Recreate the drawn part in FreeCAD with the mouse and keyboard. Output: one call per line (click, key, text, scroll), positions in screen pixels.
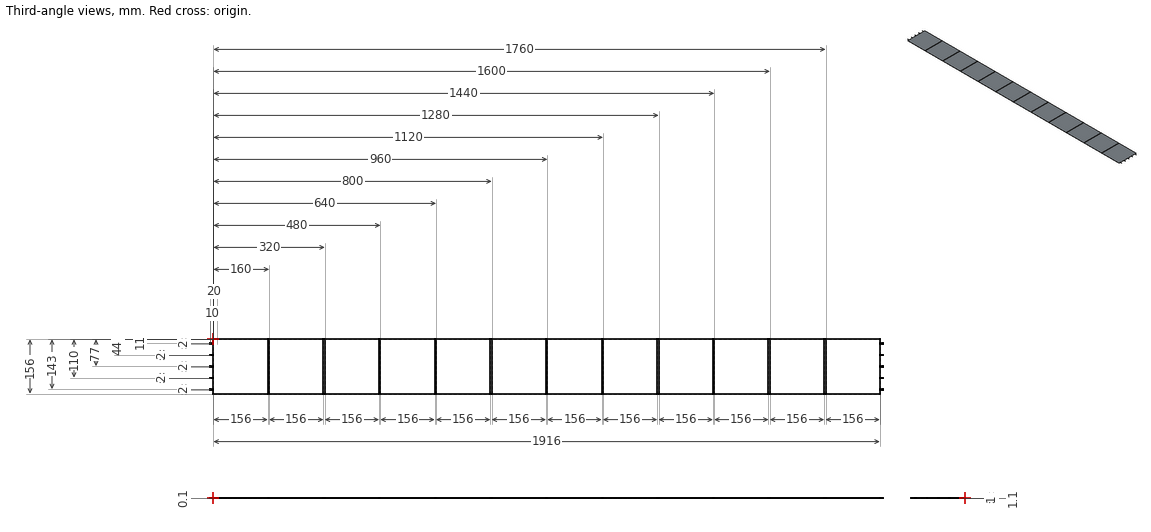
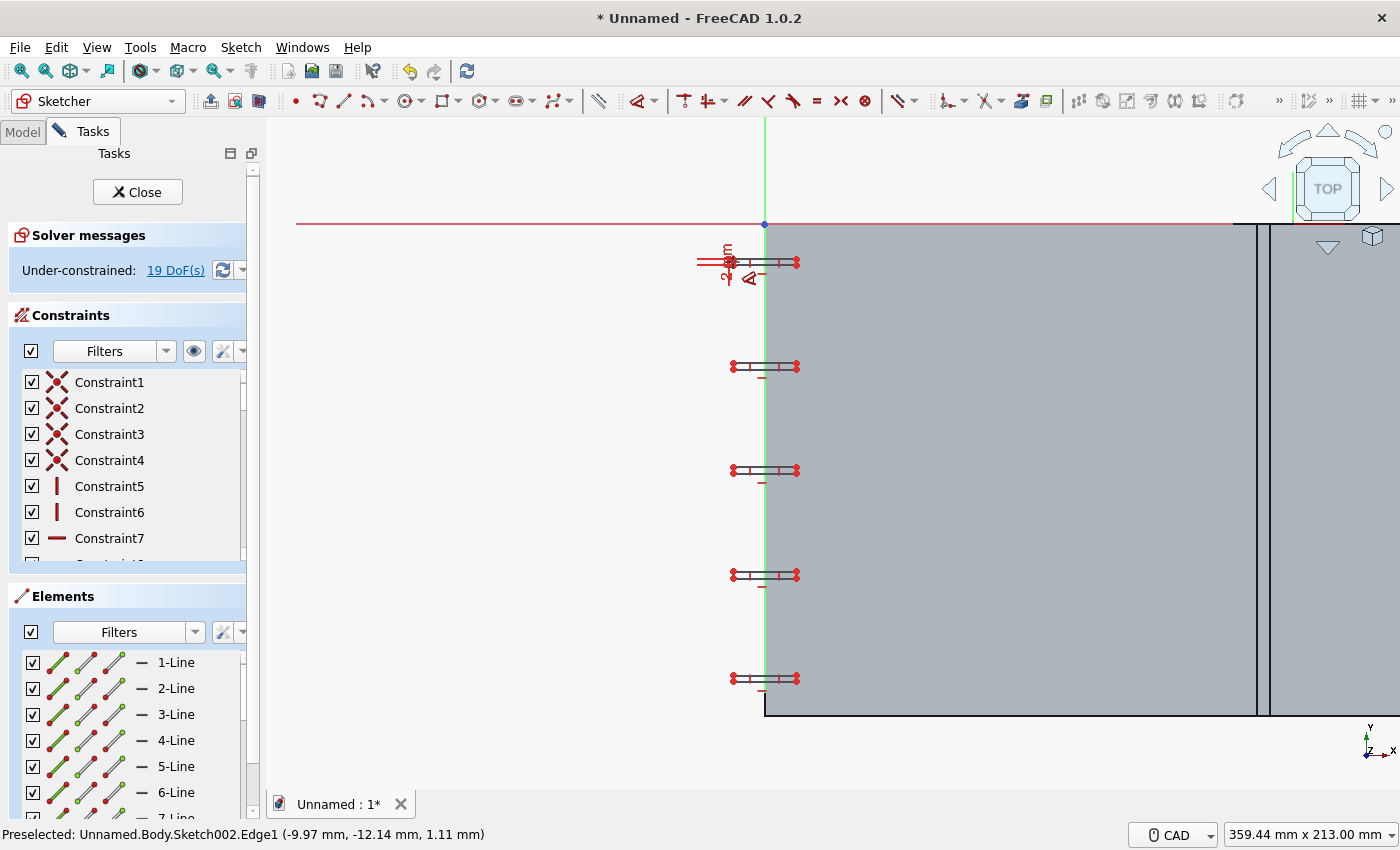
scroll(733, 365, up, 10)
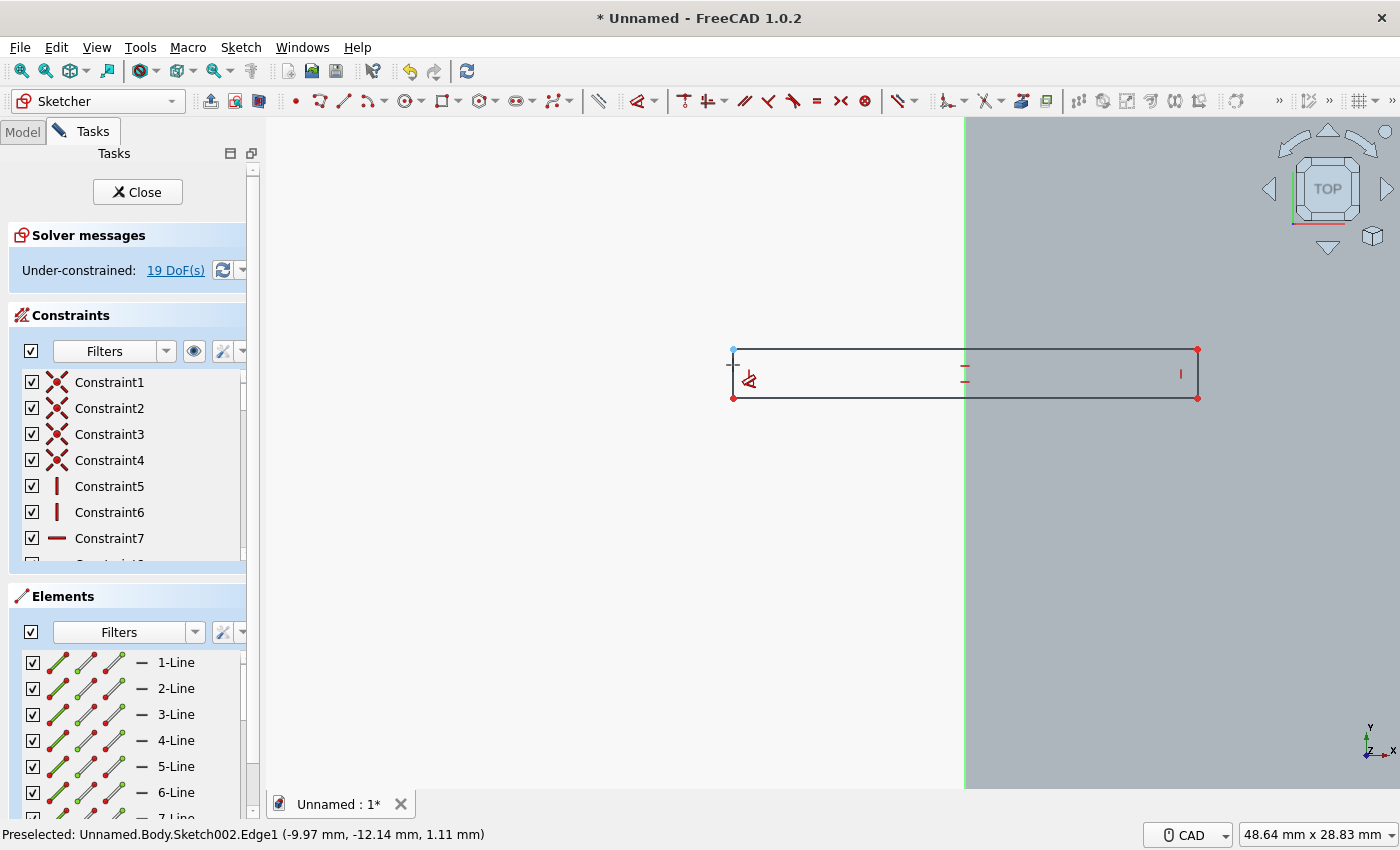
click(733, 364)
click(699, 374)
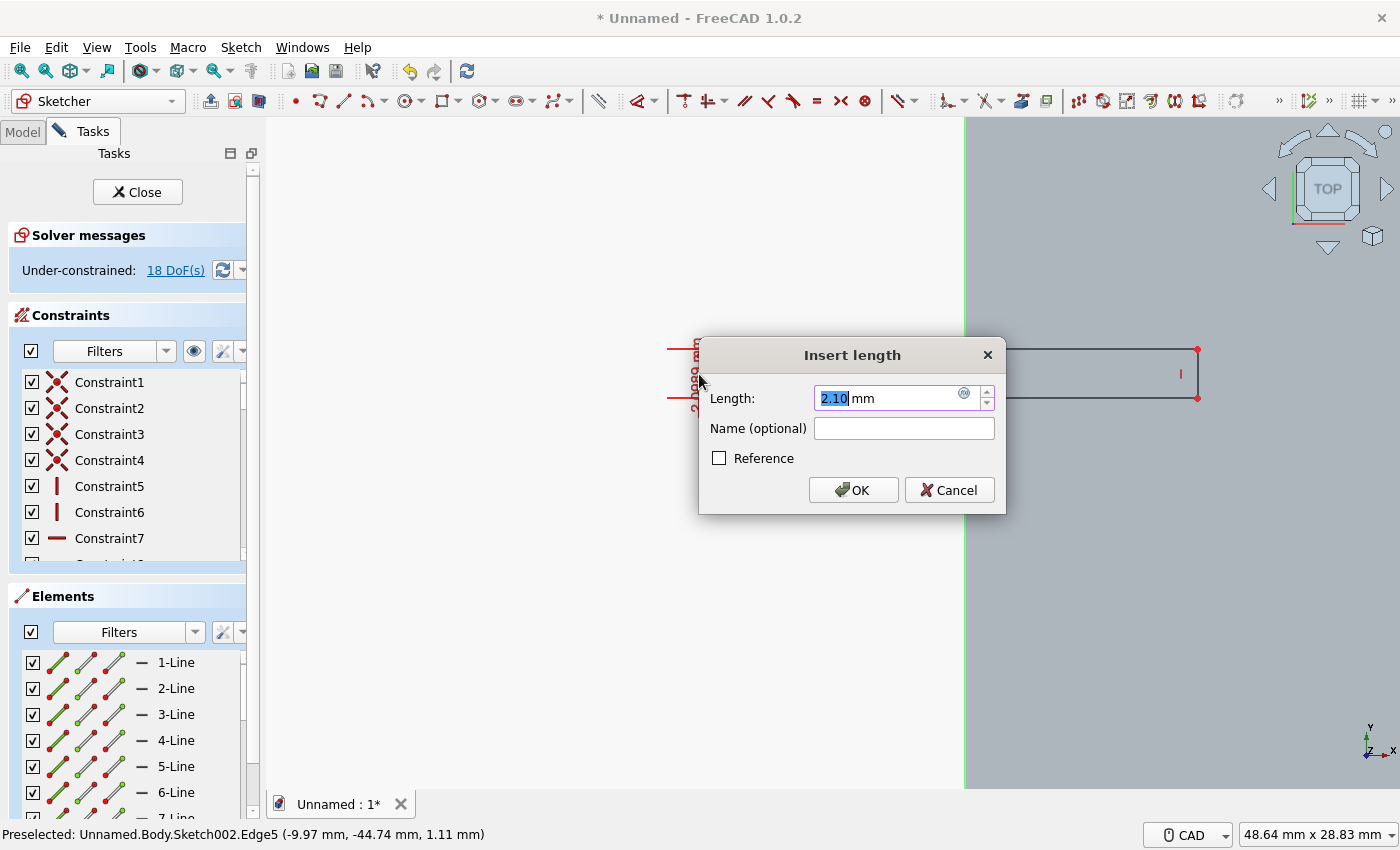
text(2)
key(Return)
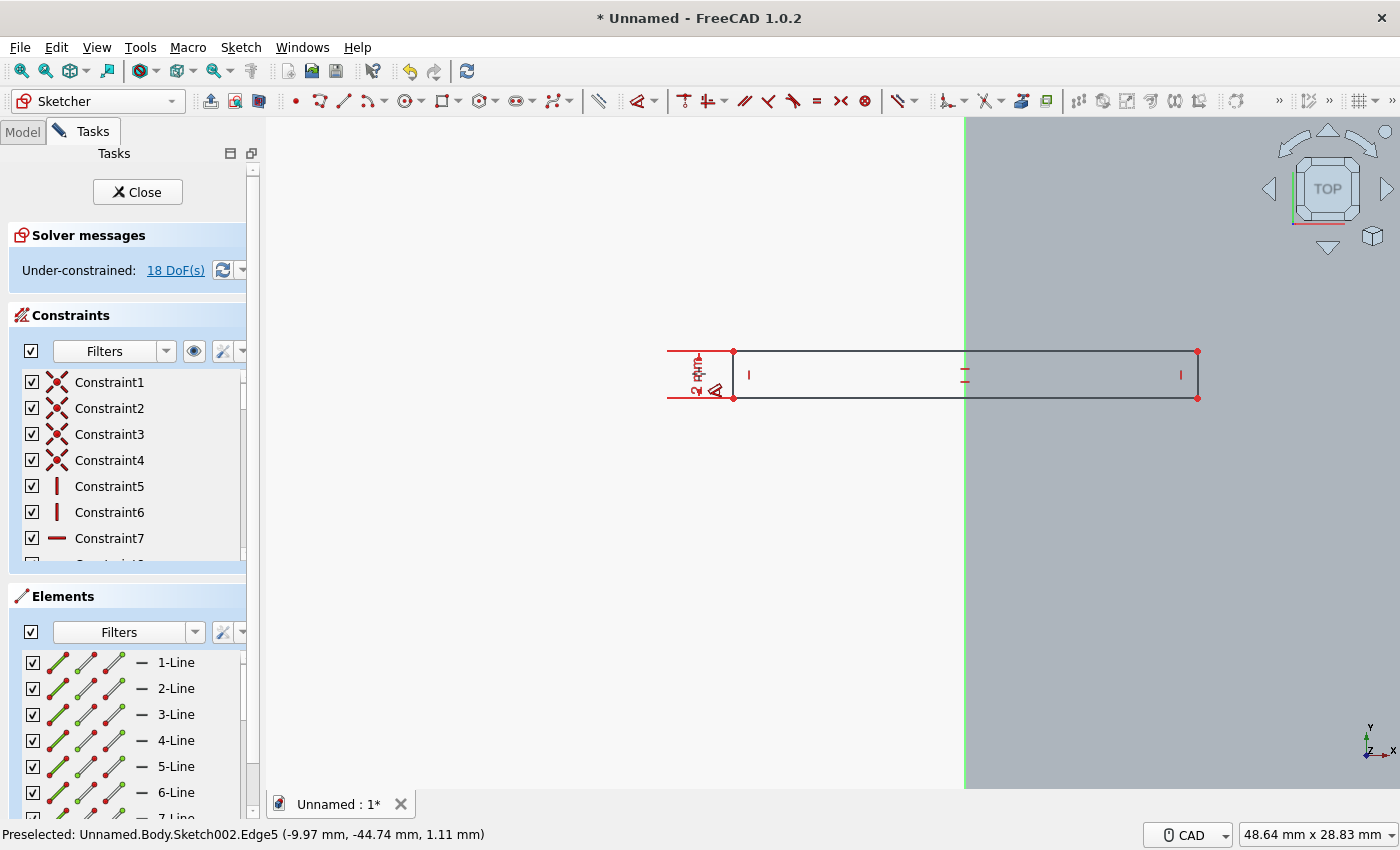
scroll(733, 365, down, 10)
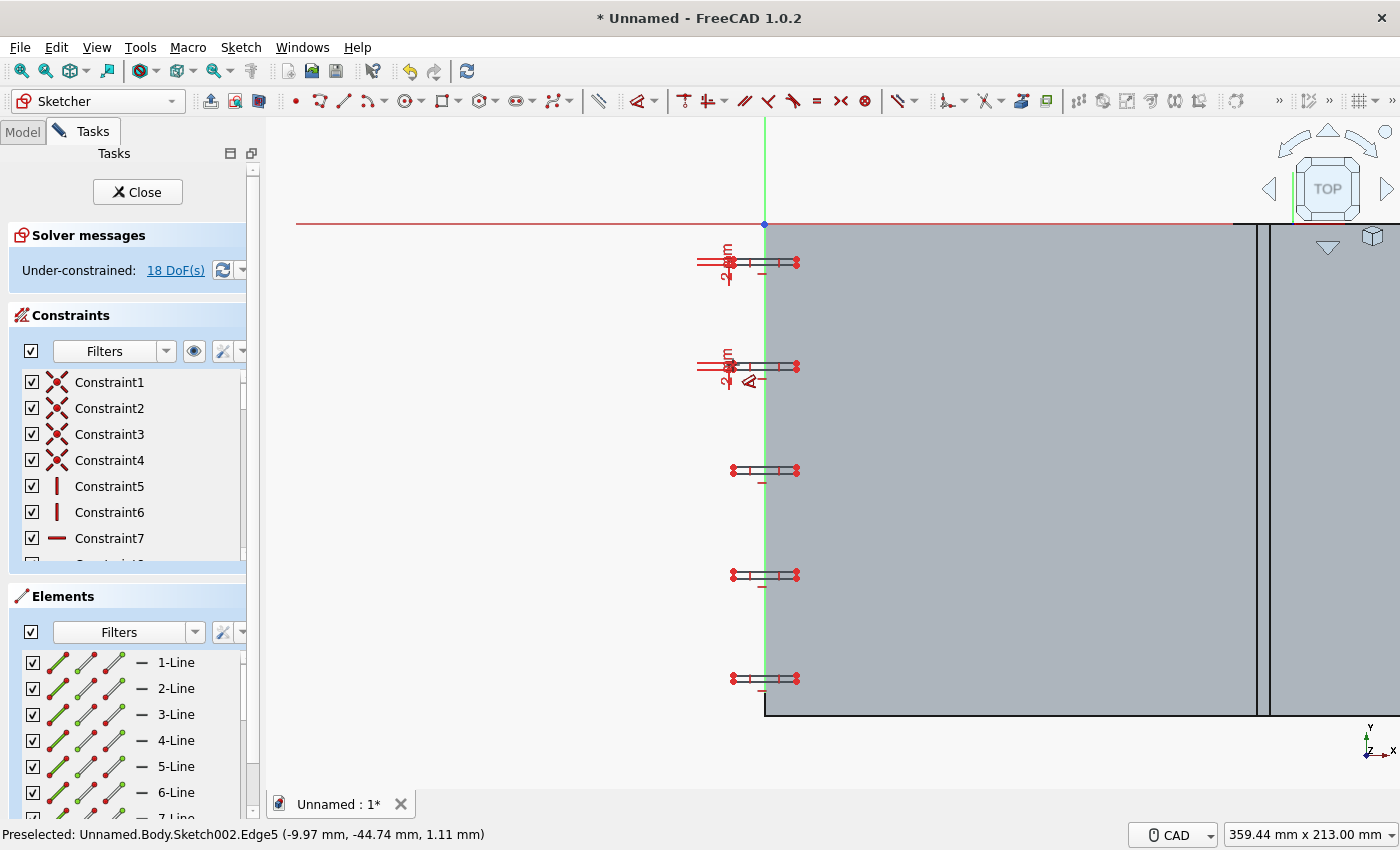
scroll(733, 469, up, 10)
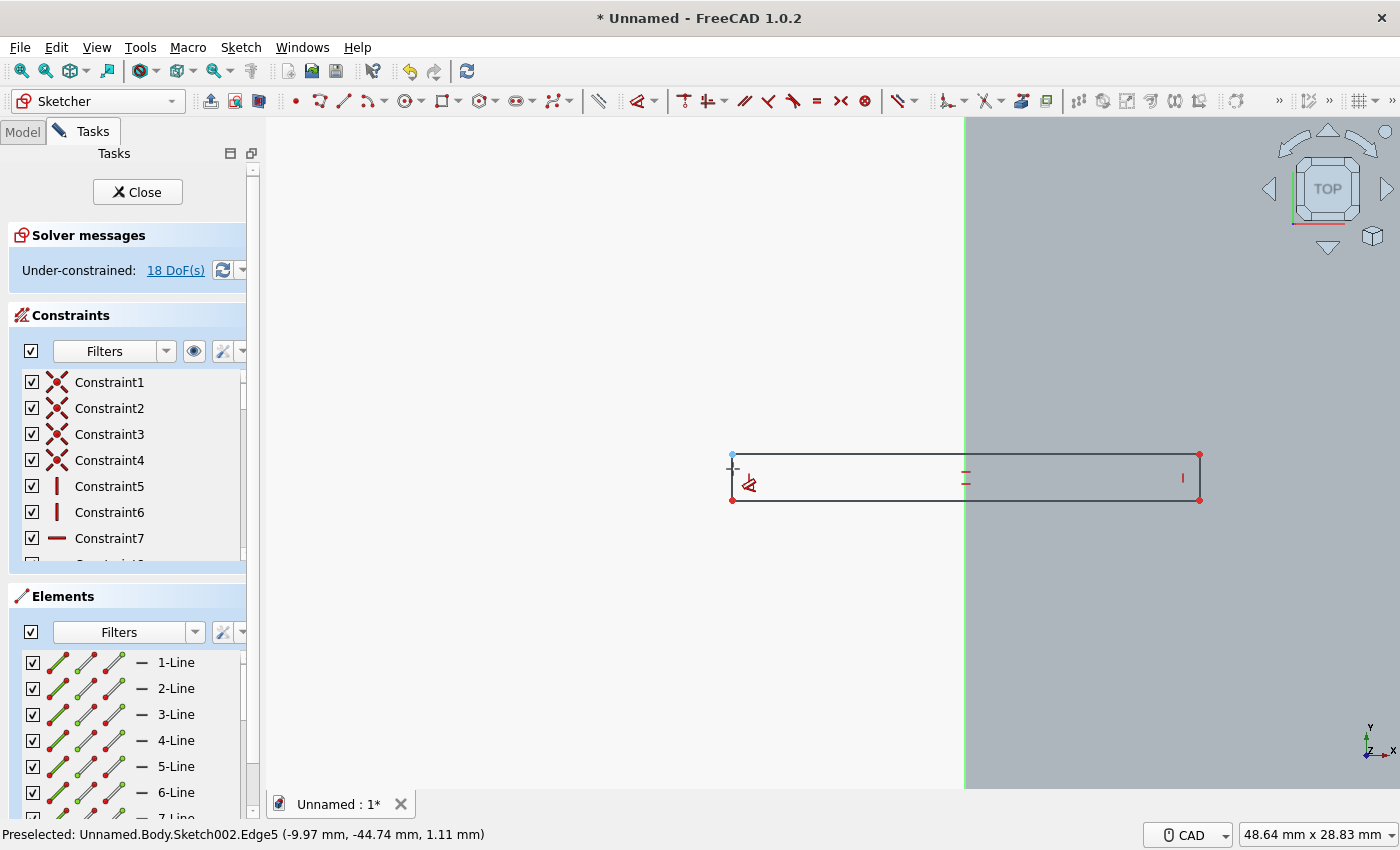
click(732, 468)
click(698, 477)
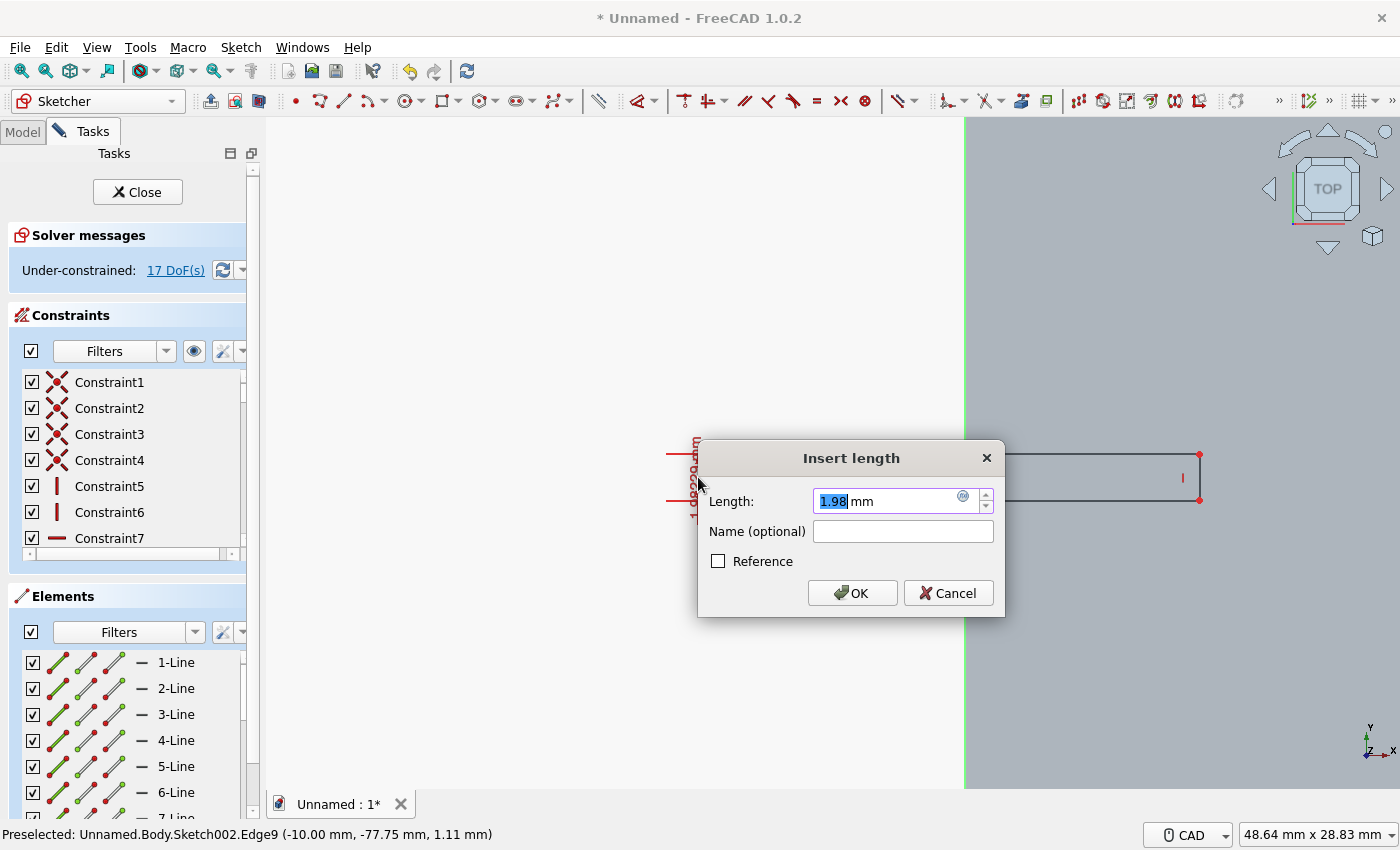
text(2)
key(Return)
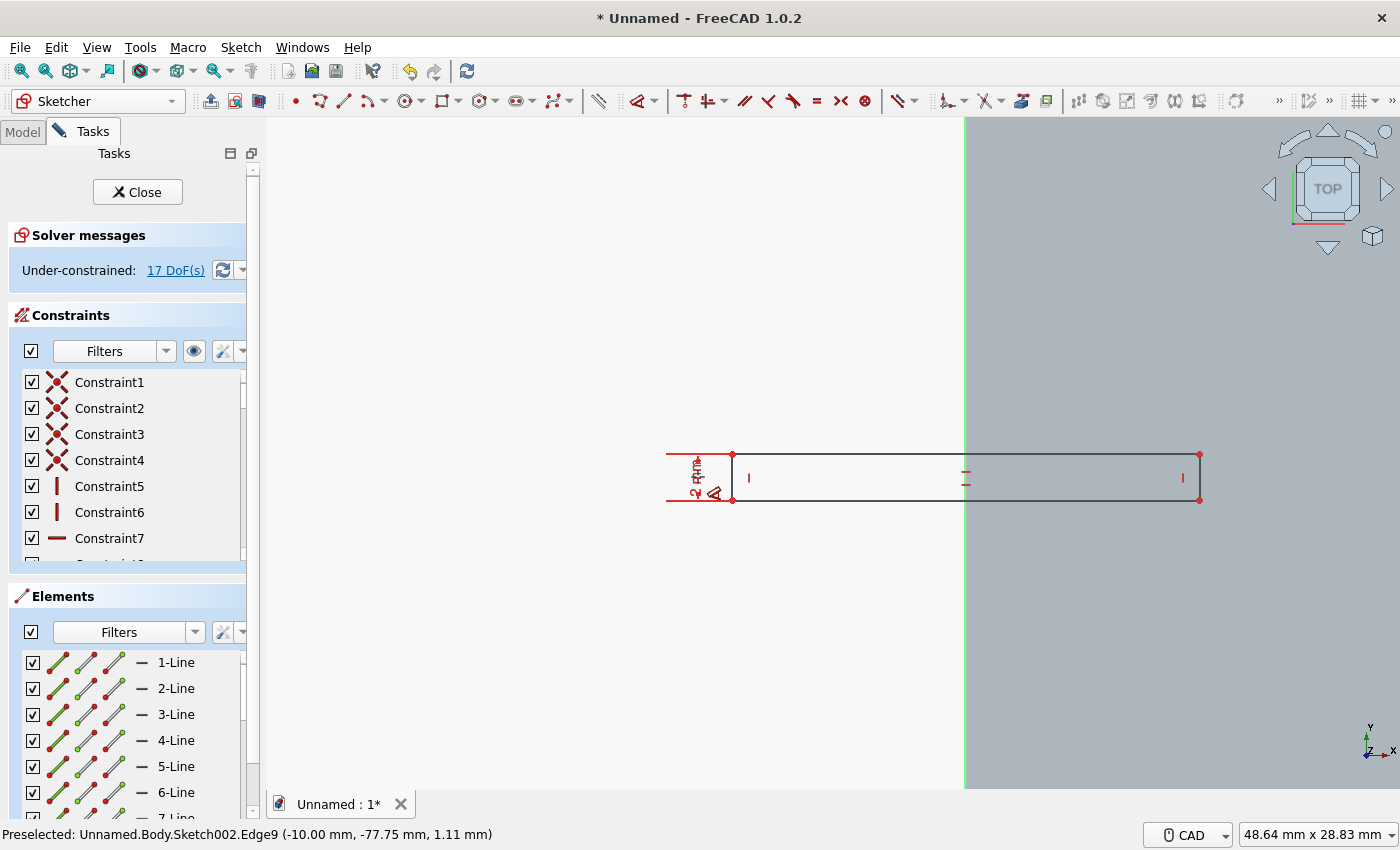
scroll(733, 470, down, 10)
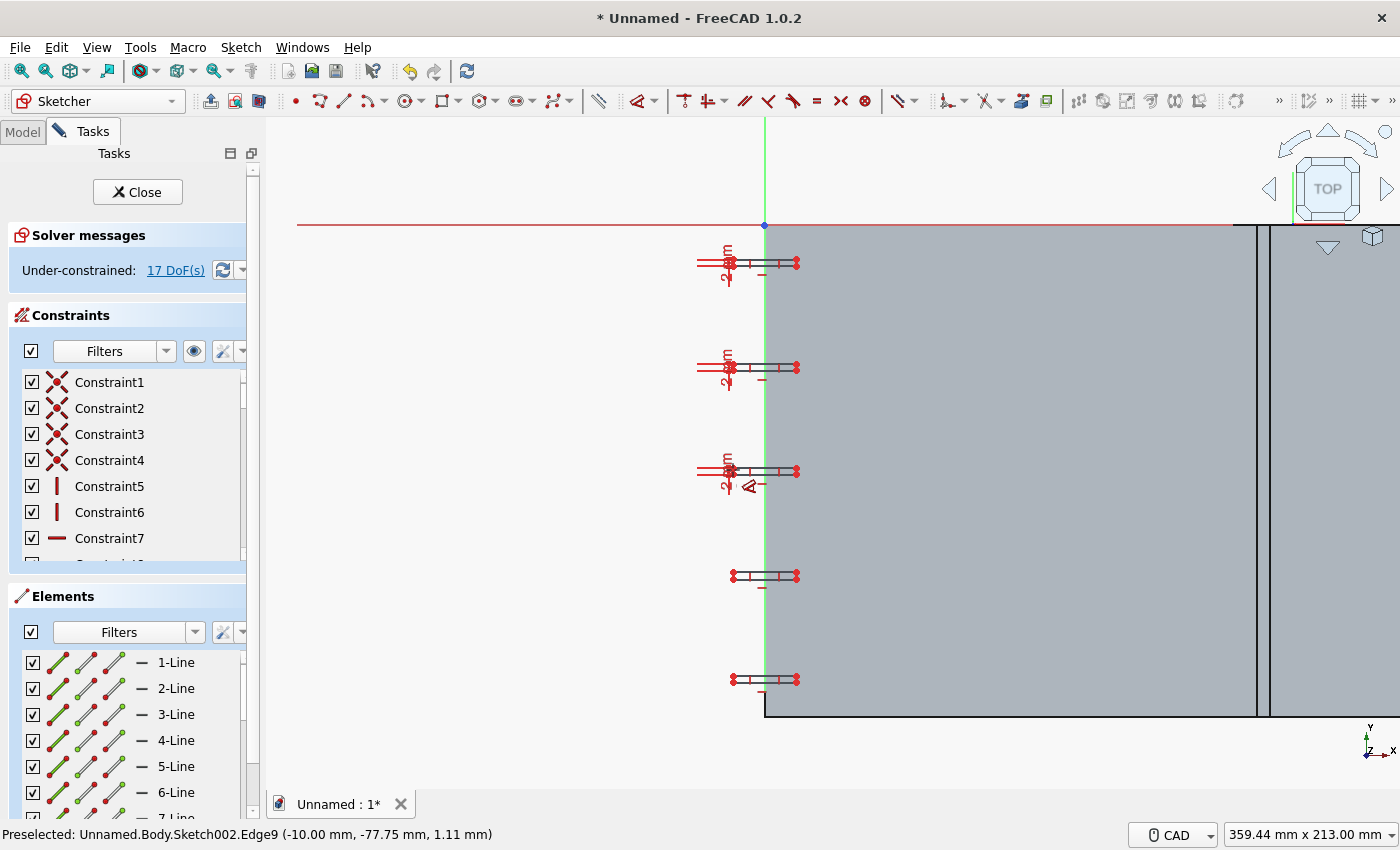
scroll(733, 575, up, 10)